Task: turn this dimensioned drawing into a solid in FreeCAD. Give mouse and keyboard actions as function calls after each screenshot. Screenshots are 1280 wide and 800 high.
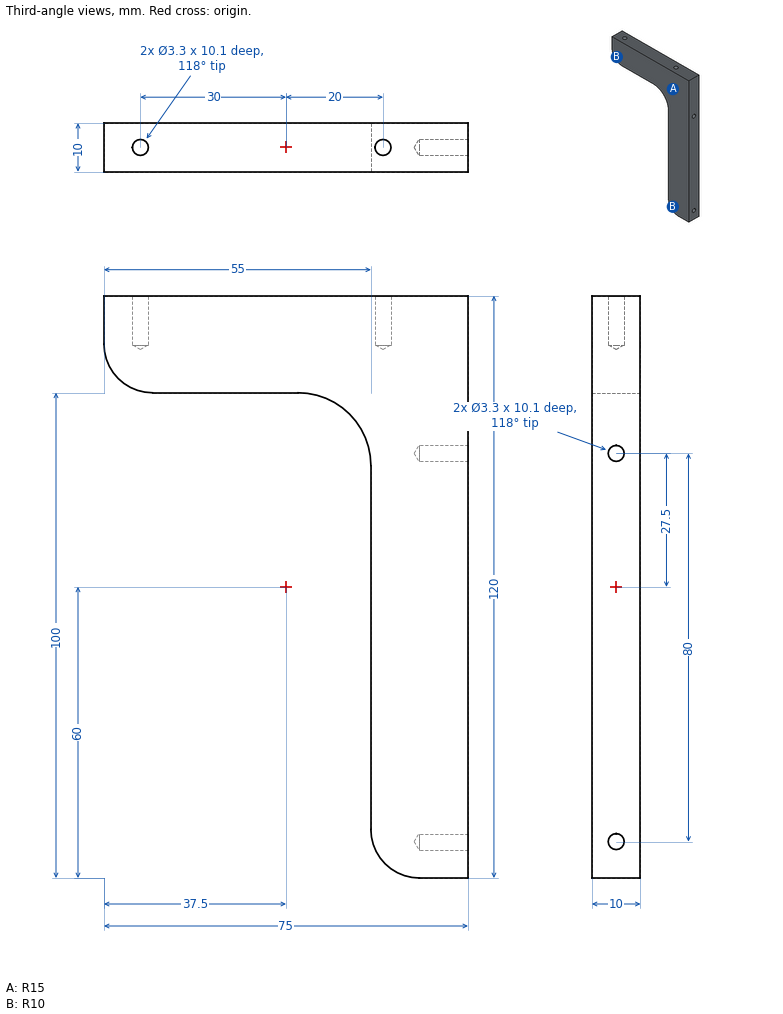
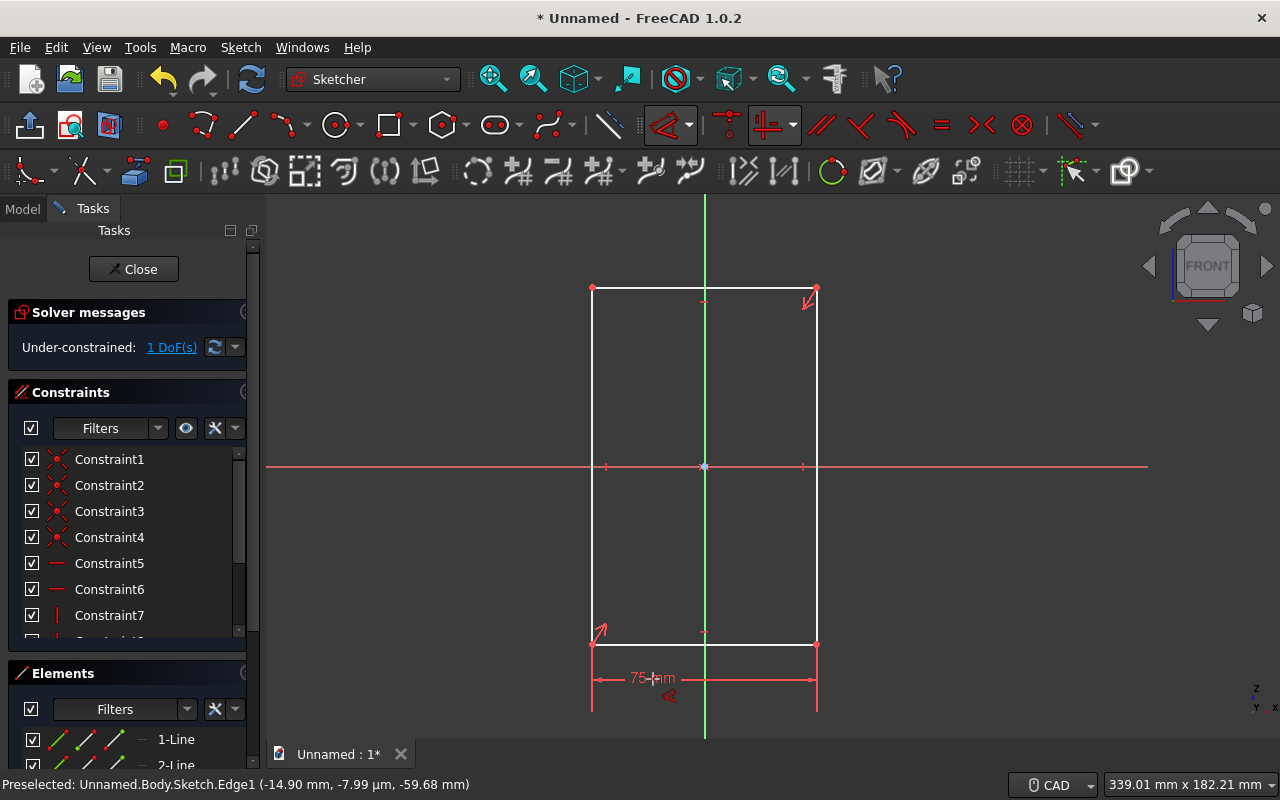
click(817, 538)
click(851, 384)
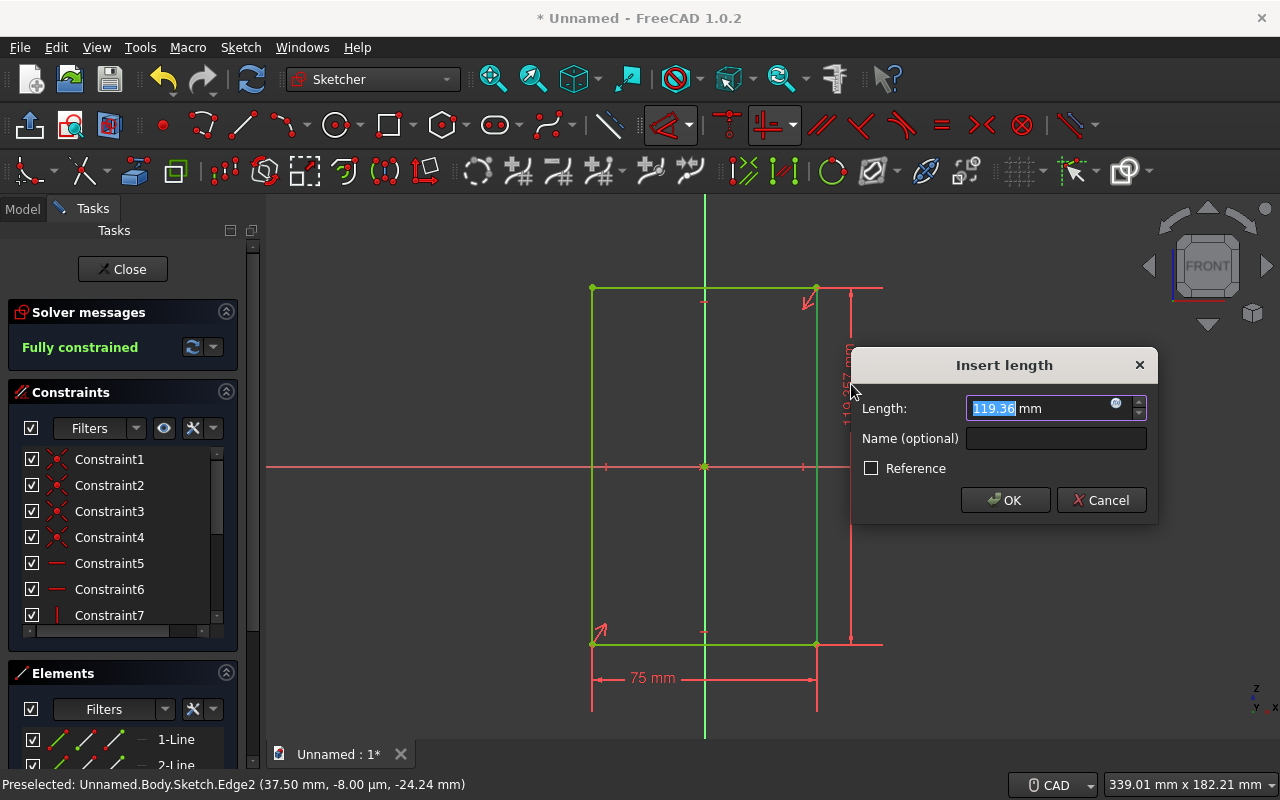
text(120)
key(Return)
key(Escape)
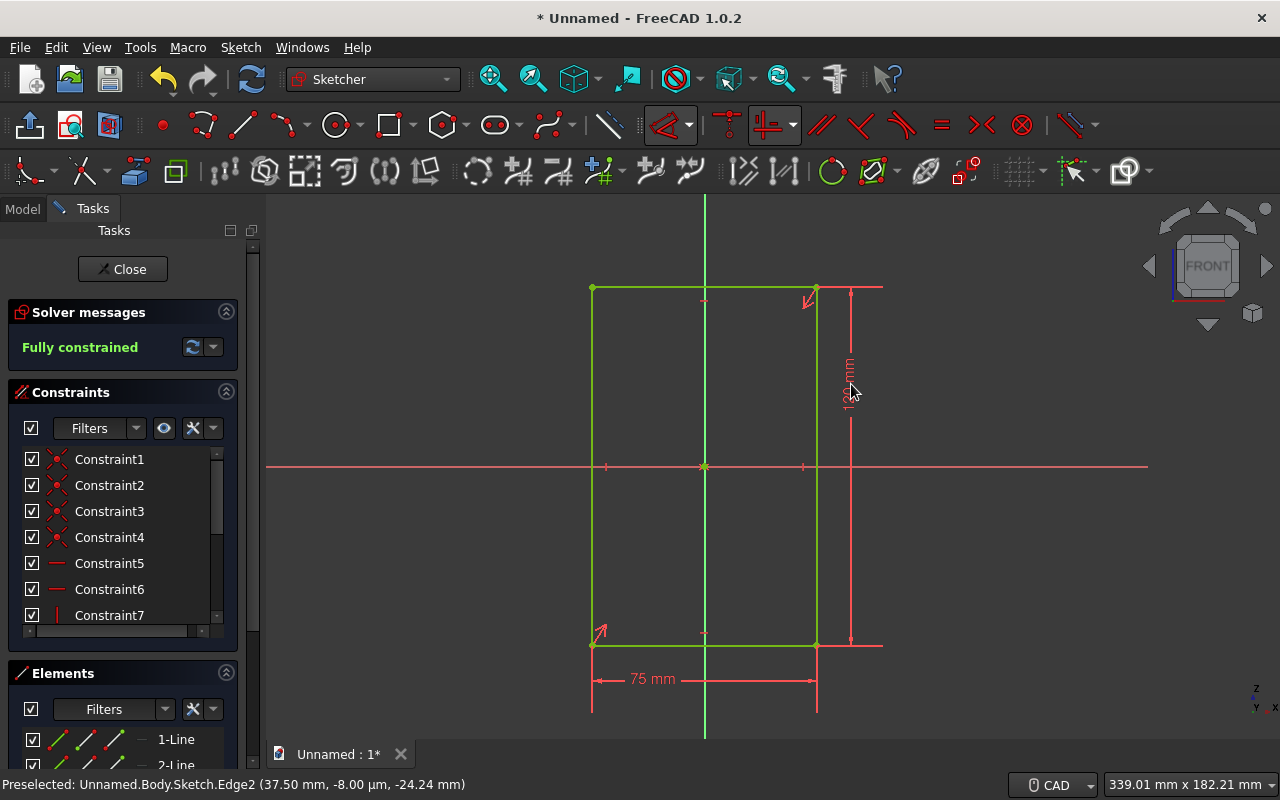
click(123, 269)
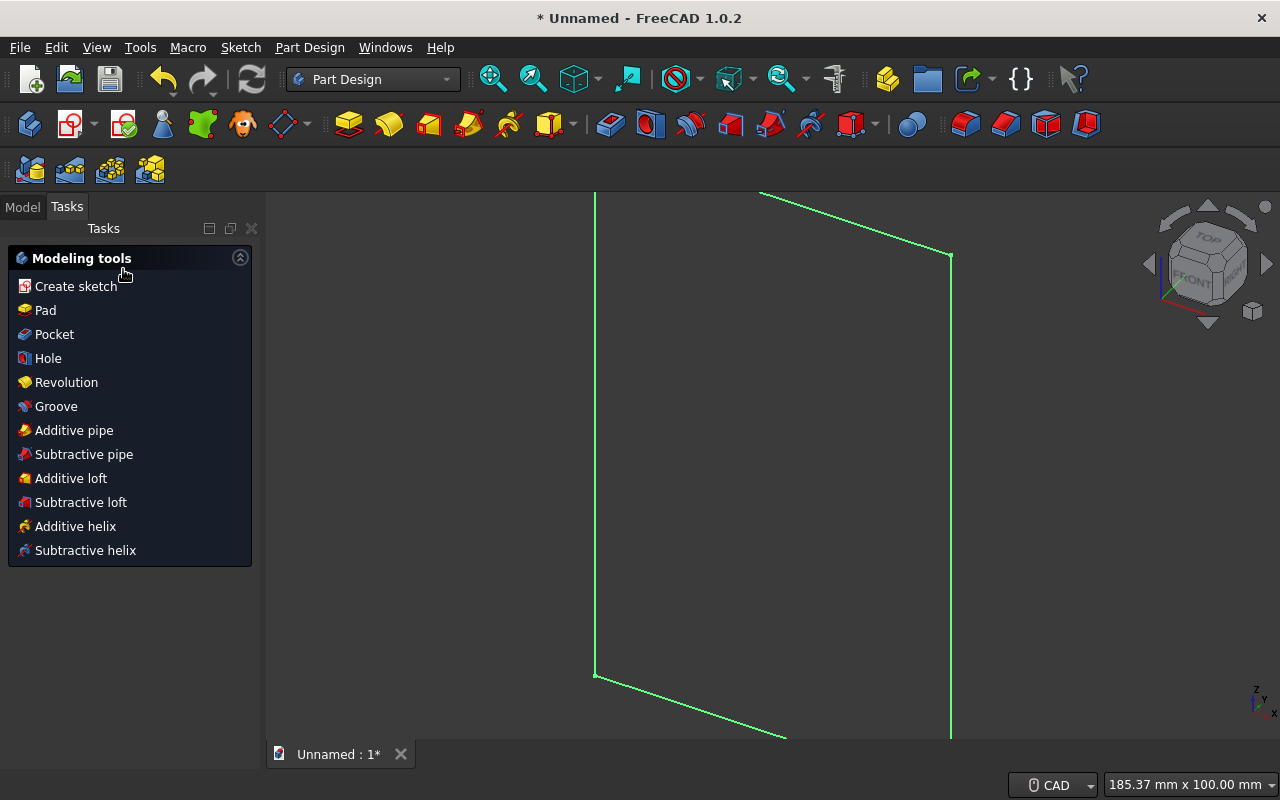
click(350, 124)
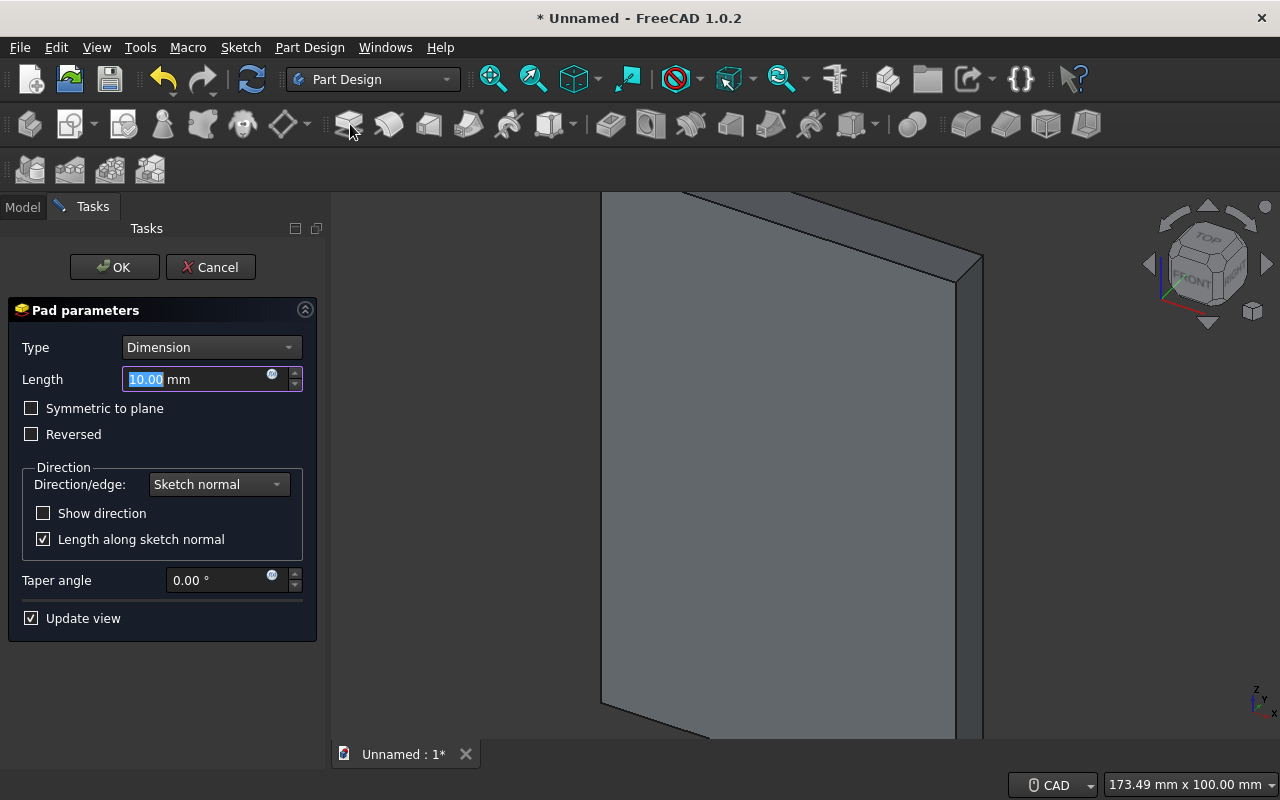
text(10)
key(Tab)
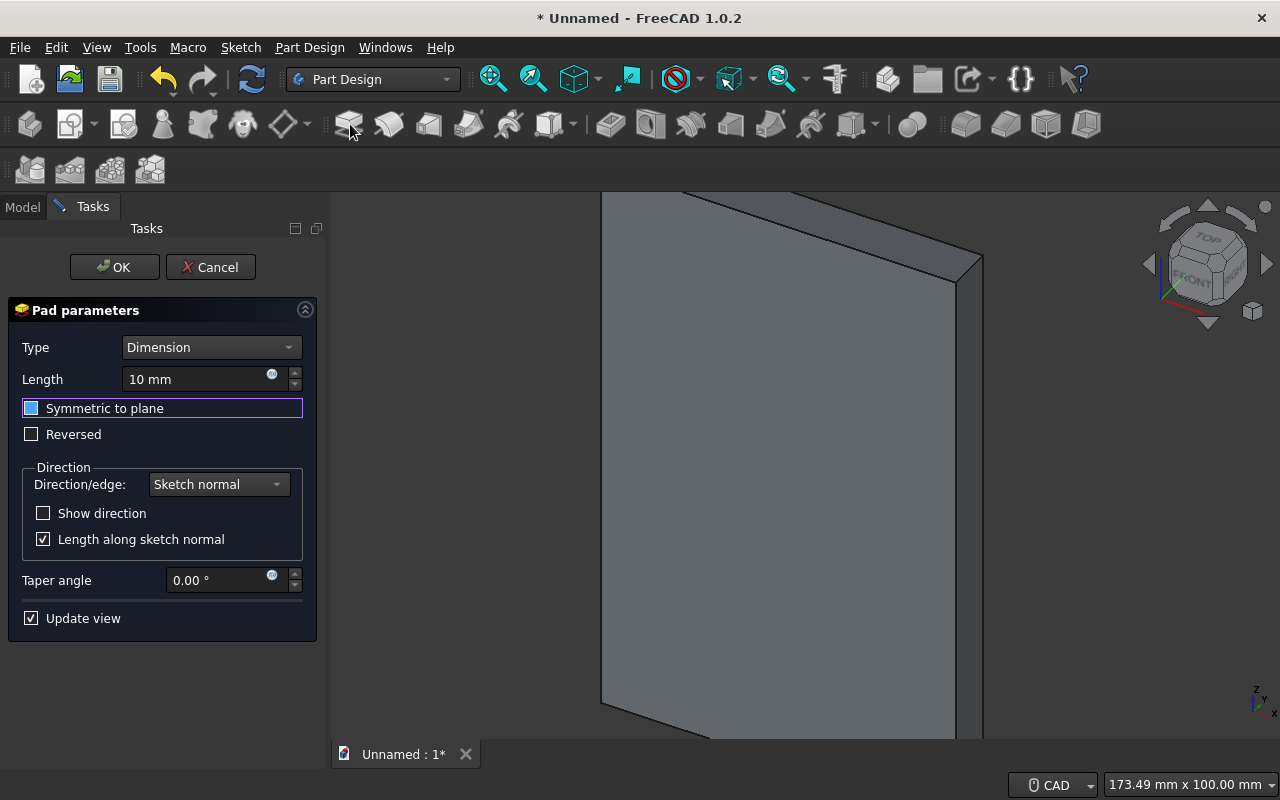
click(30, 408)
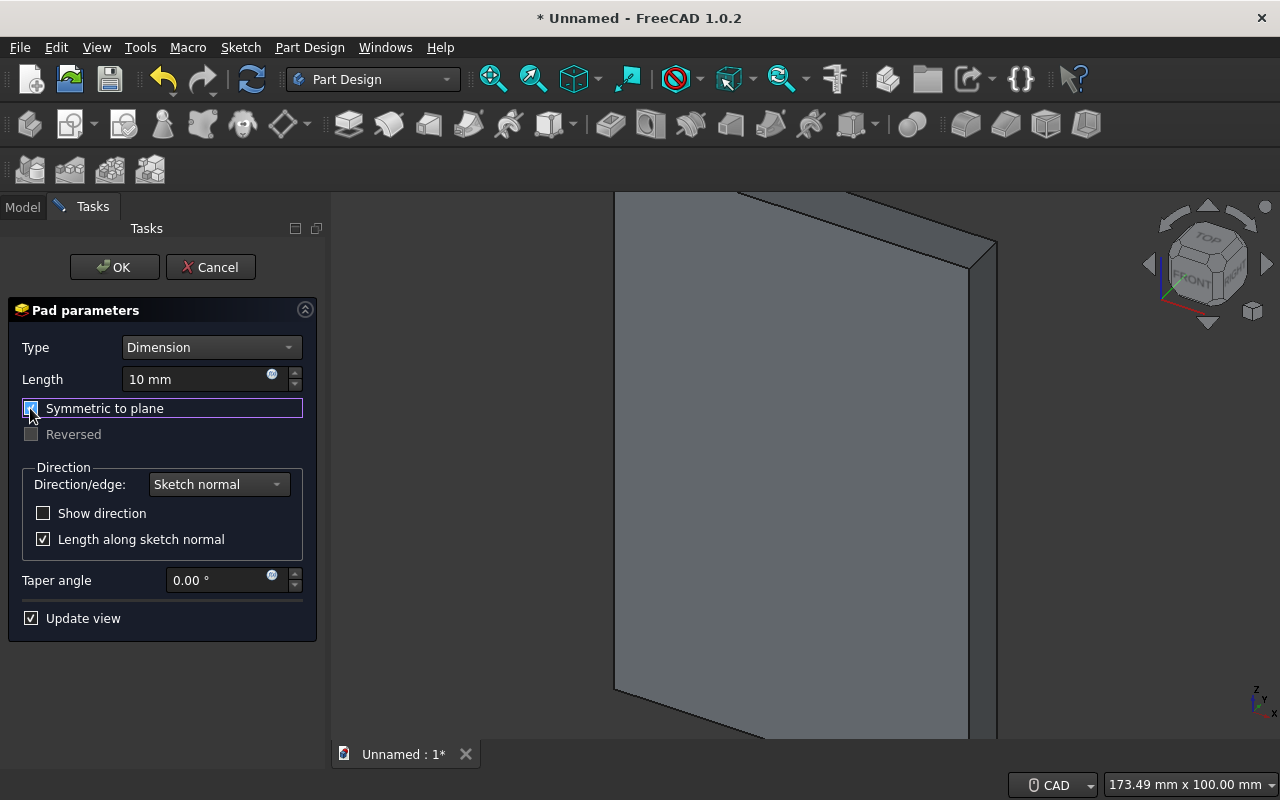
click(115, 267)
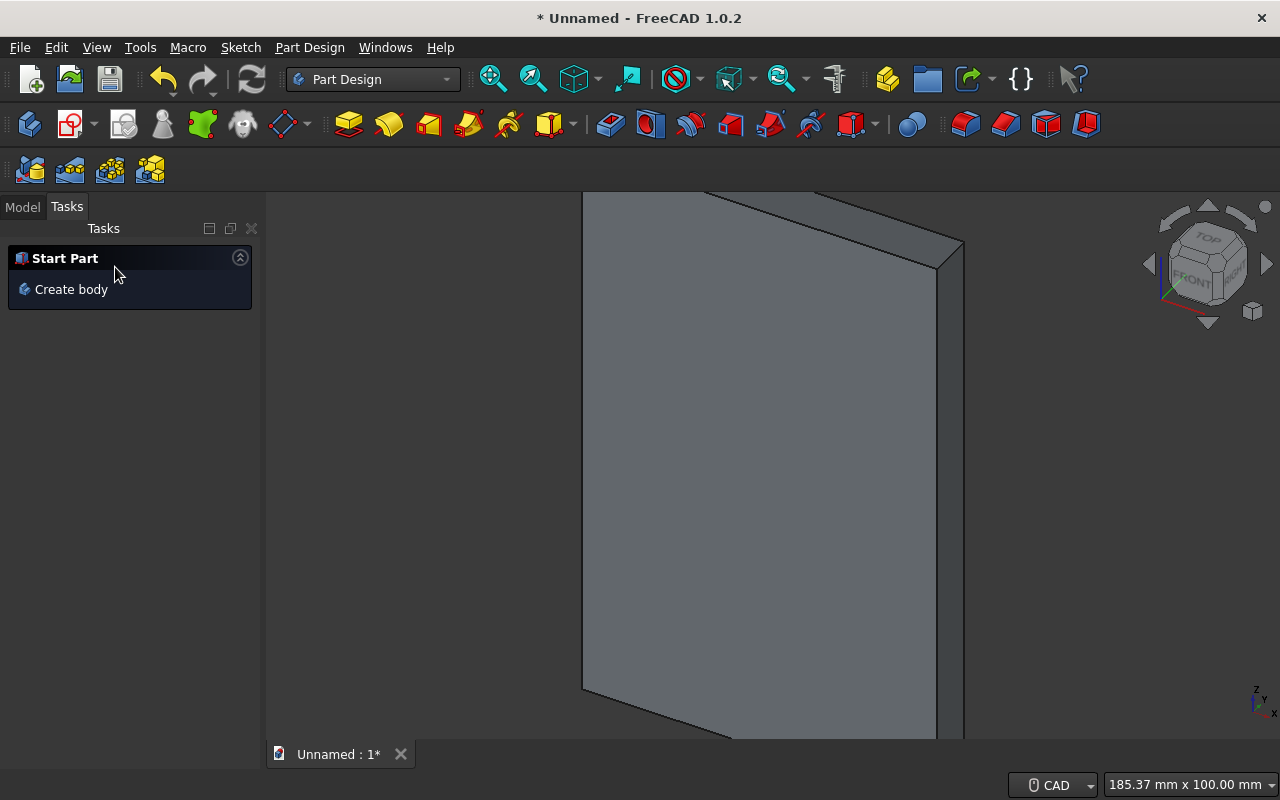
key(v)
key(f)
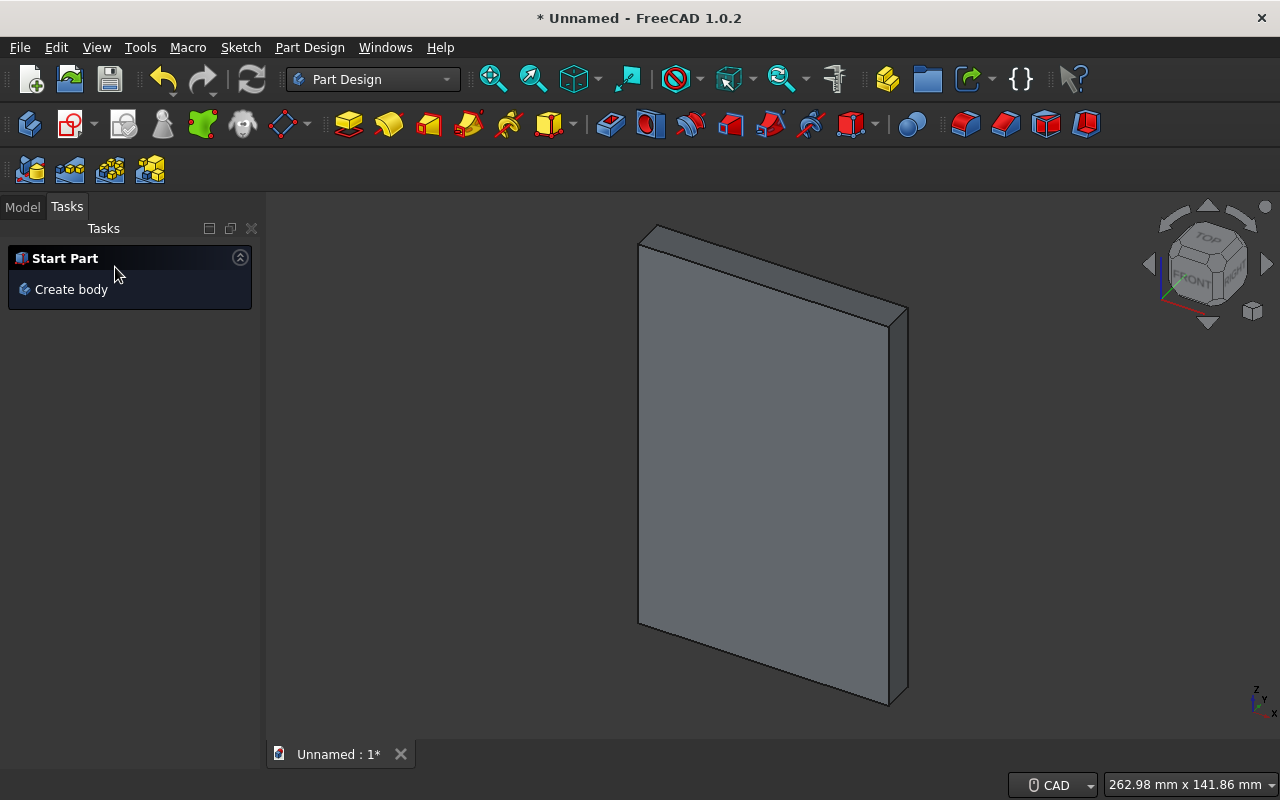
key(4)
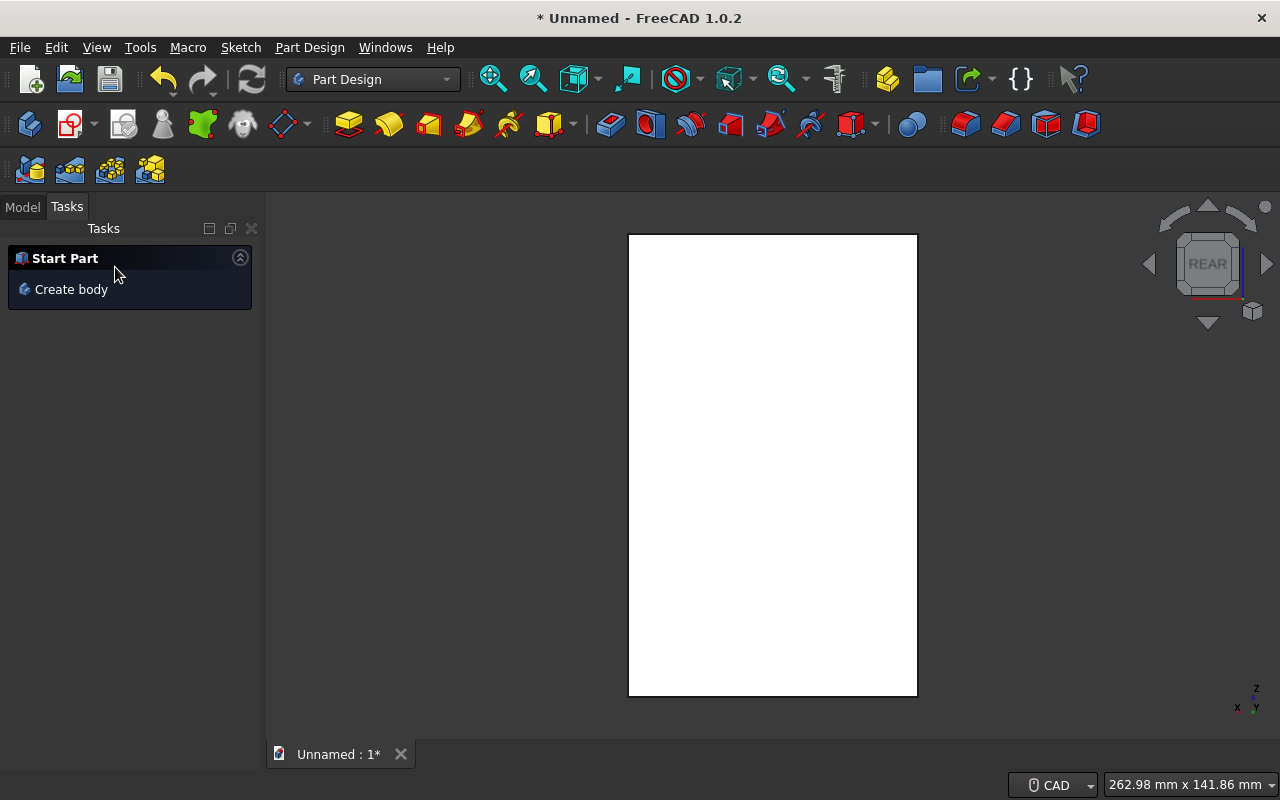
click(773, 398)